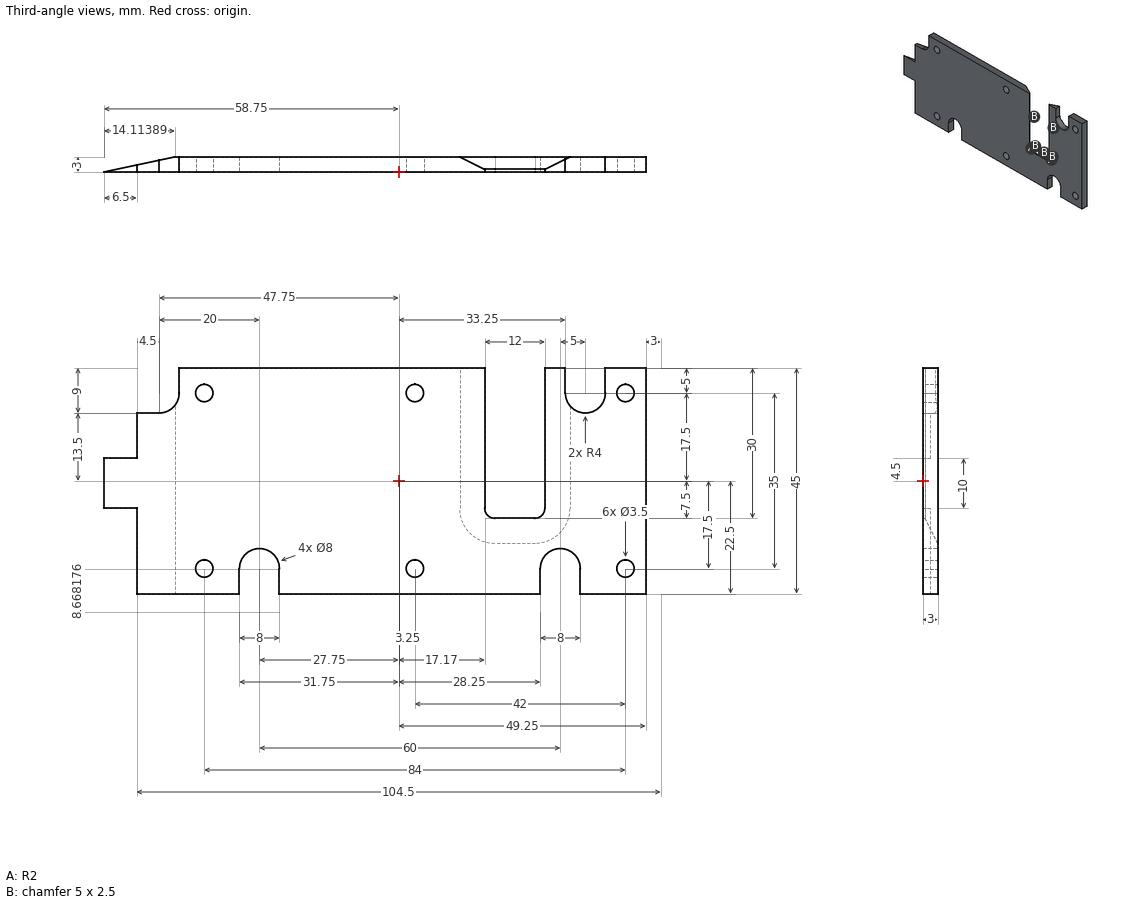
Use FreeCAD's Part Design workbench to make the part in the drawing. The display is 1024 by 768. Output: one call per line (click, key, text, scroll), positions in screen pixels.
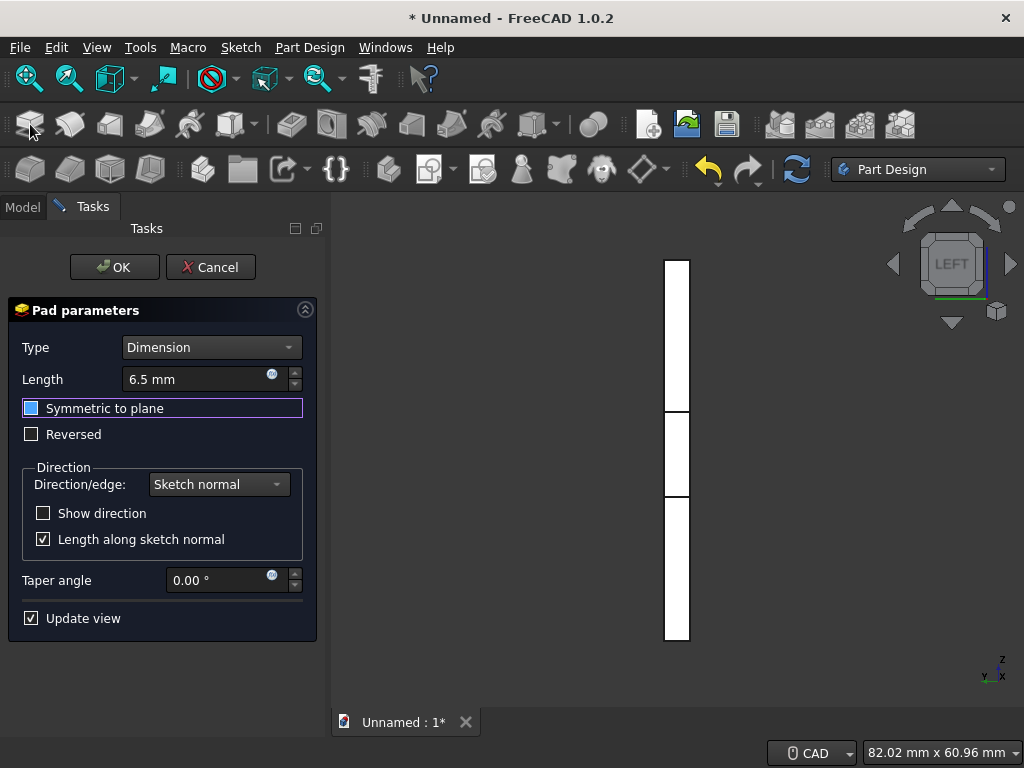
click(115, 267)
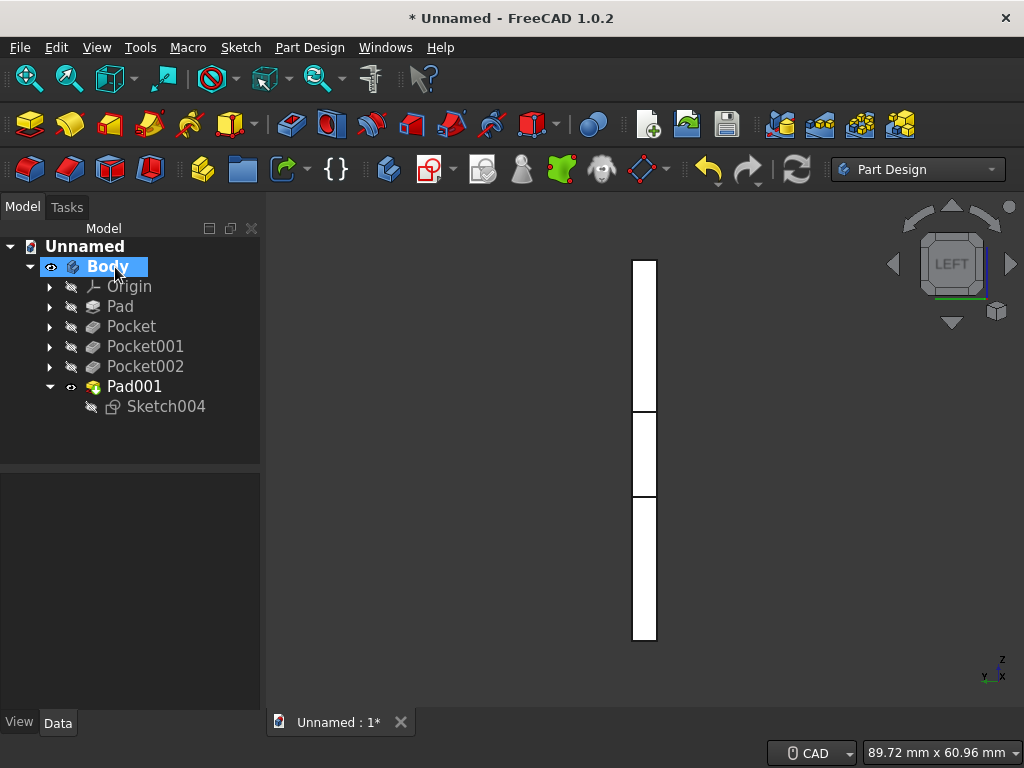
key(0)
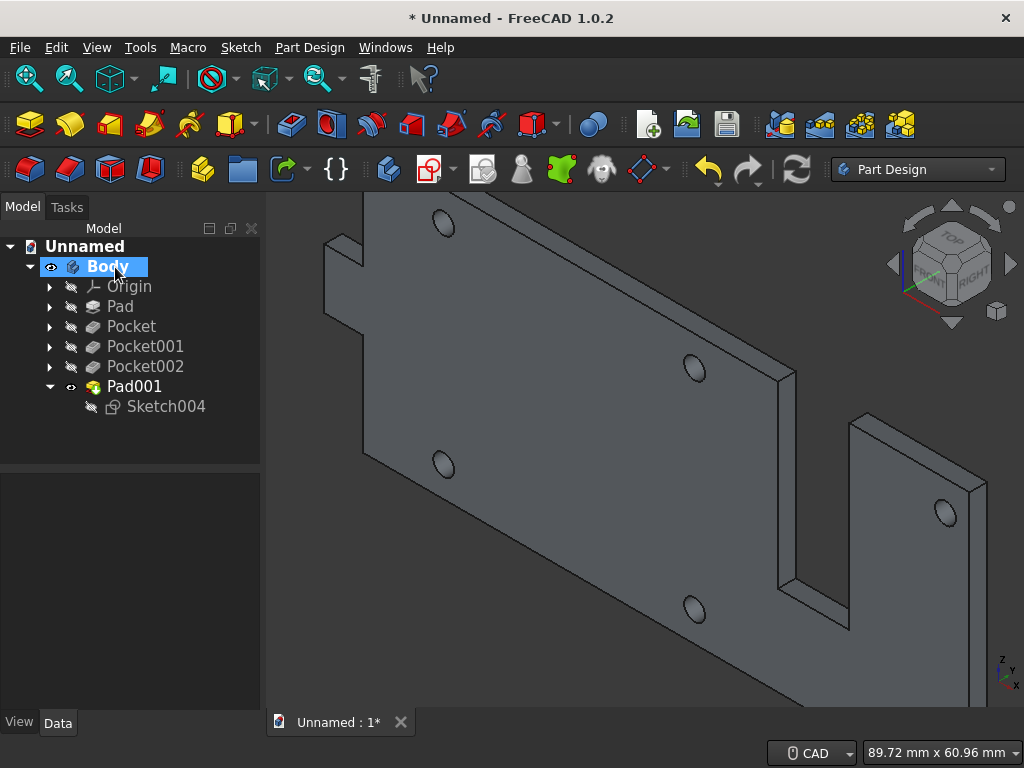
key(v)
key(f)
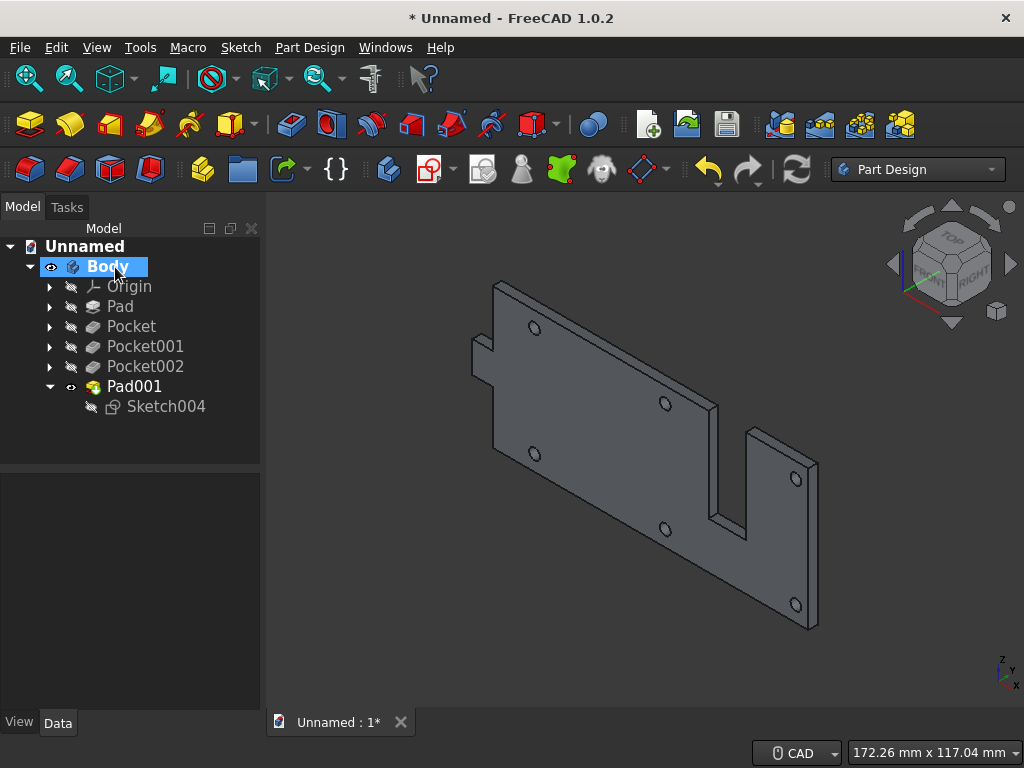
scroll(698, 398, up, 3)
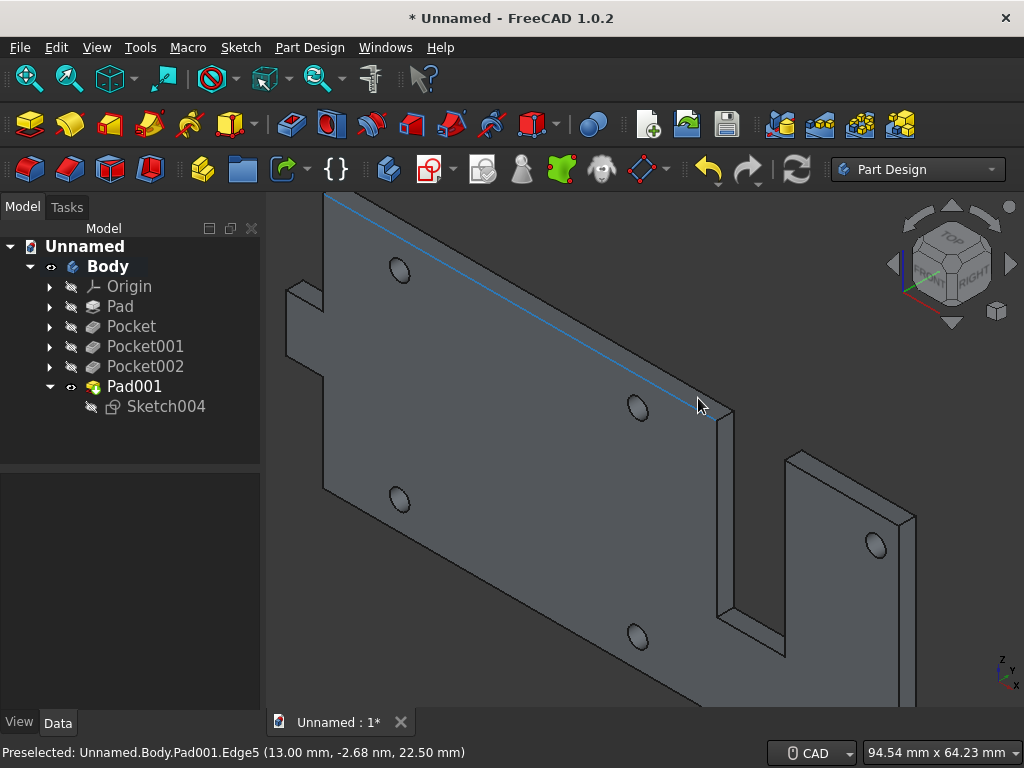
click(700, 397)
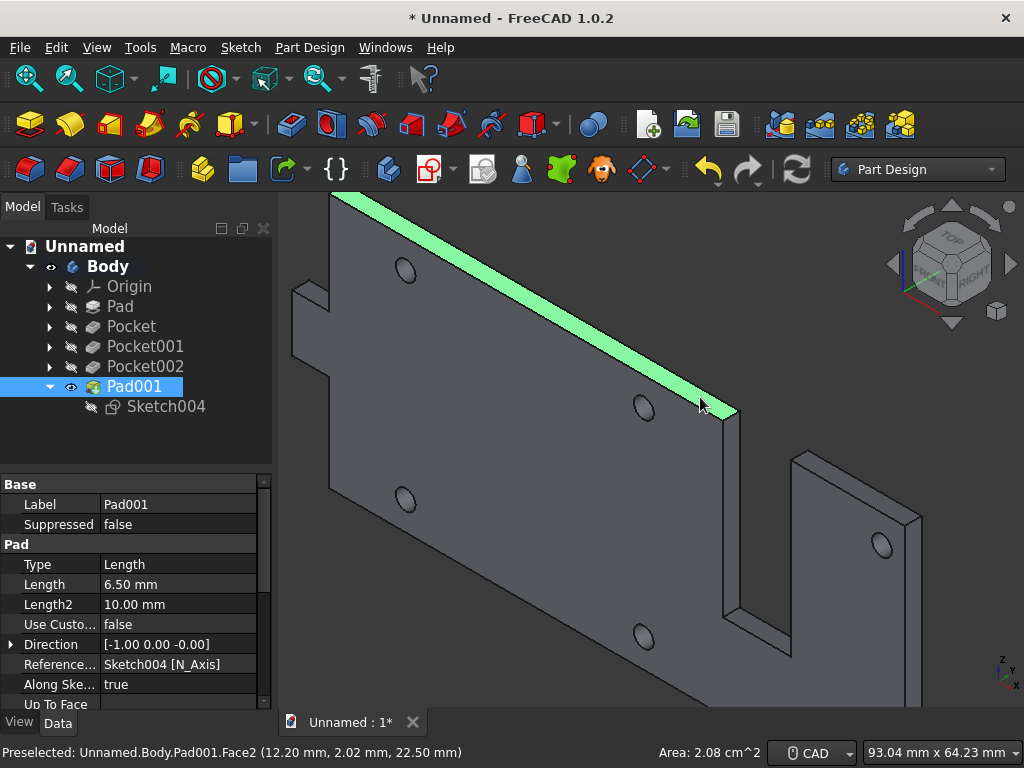
click(430, 170)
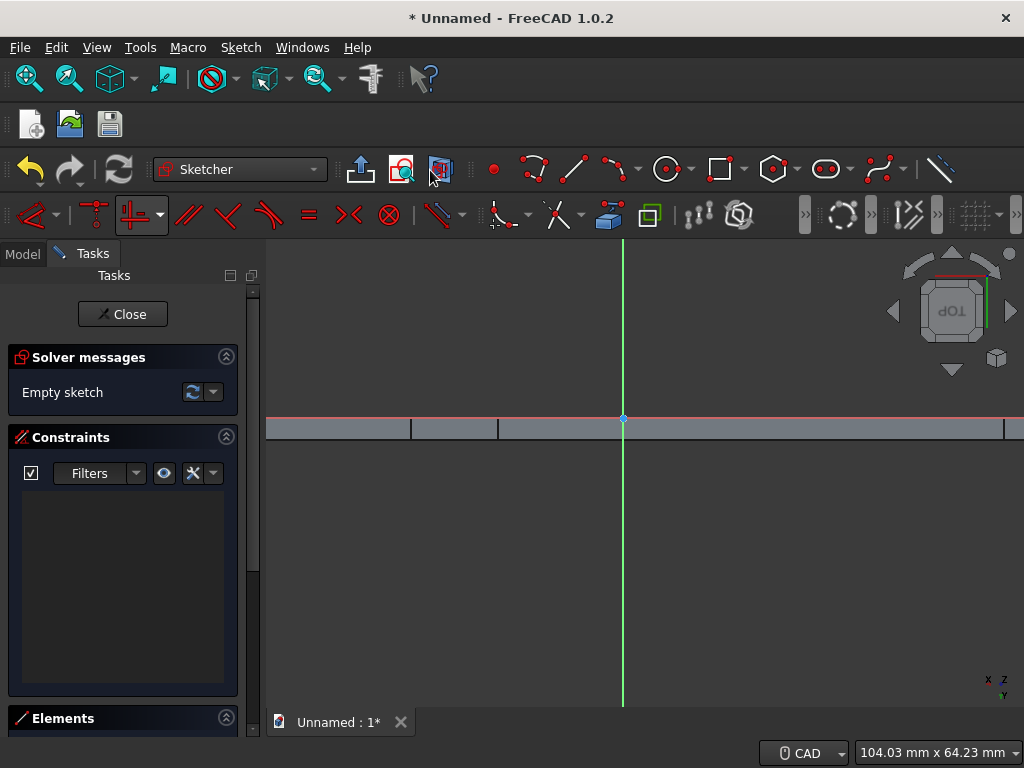
scroll(576, 473, down, 5)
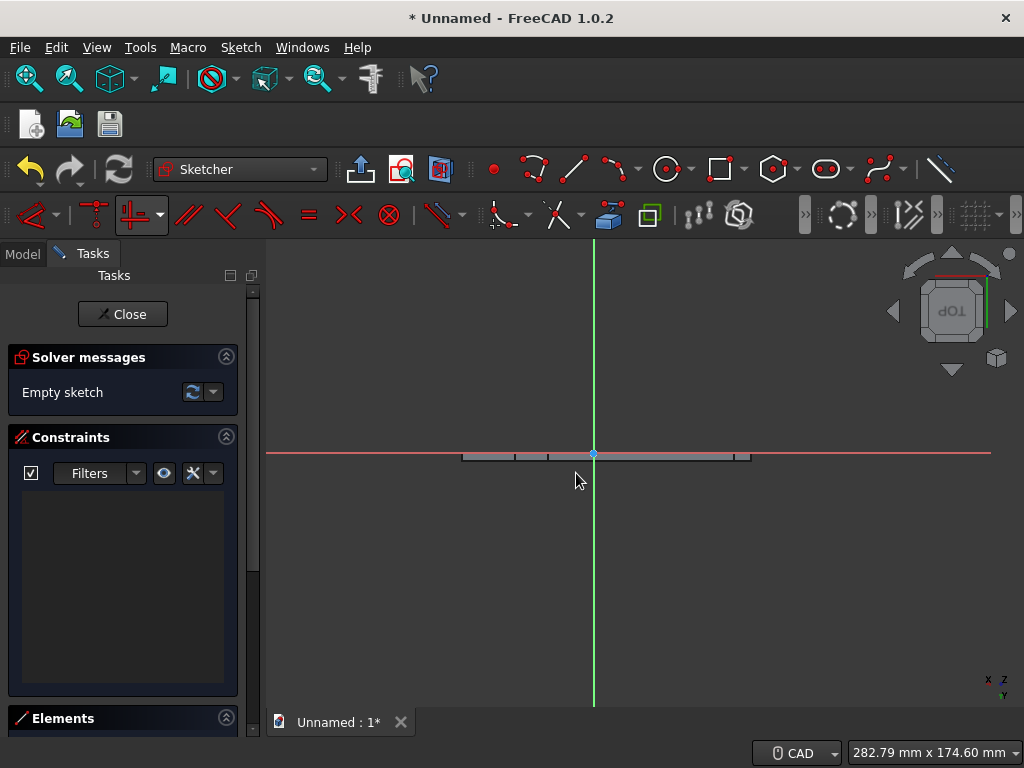
scroll(748, 456, up, 12)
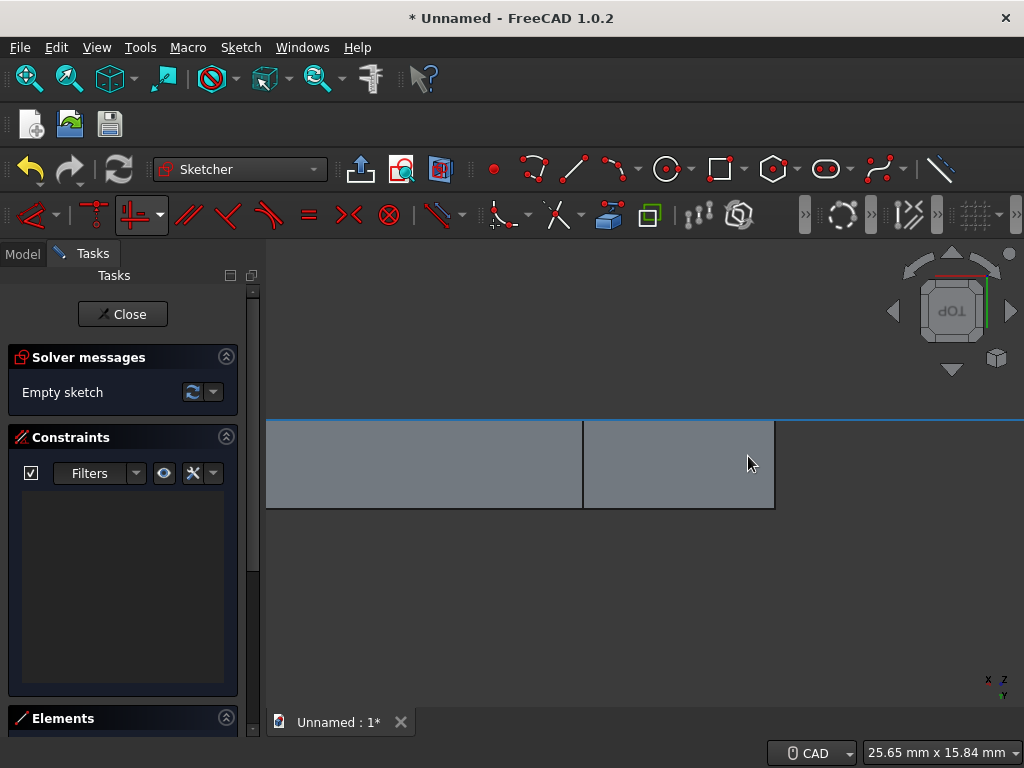
key(g)
key(m)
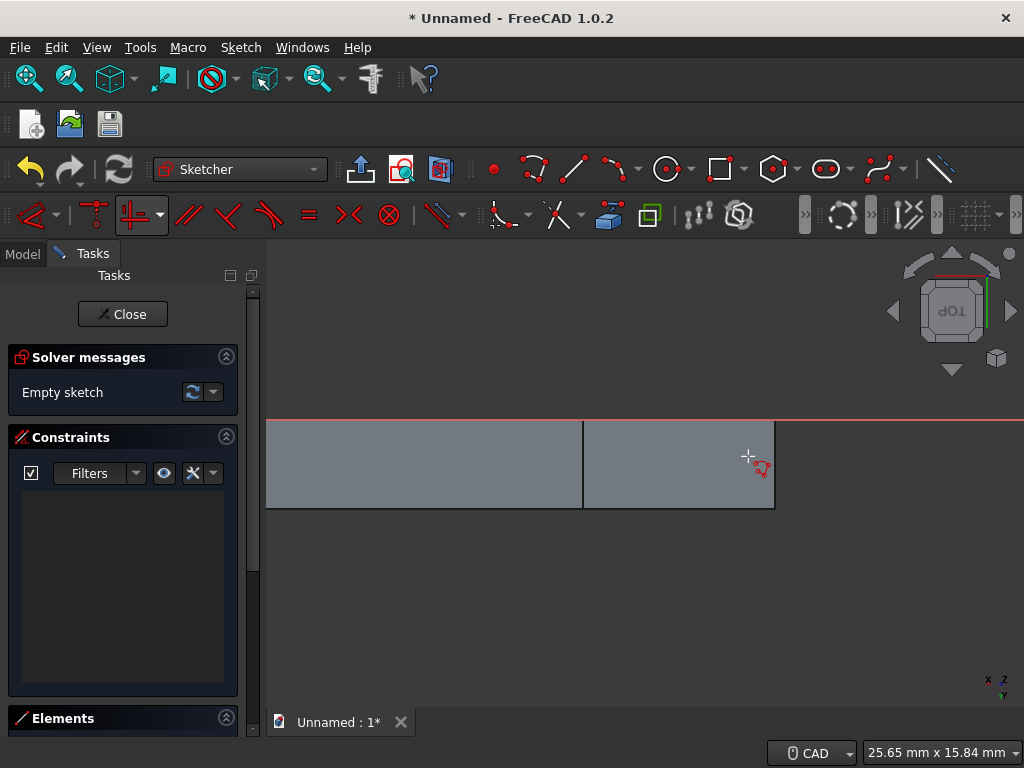
click(358, 509)
click(775, 509)
click(775, 420)
click(358, 510)
key(Escape)
key(Escape)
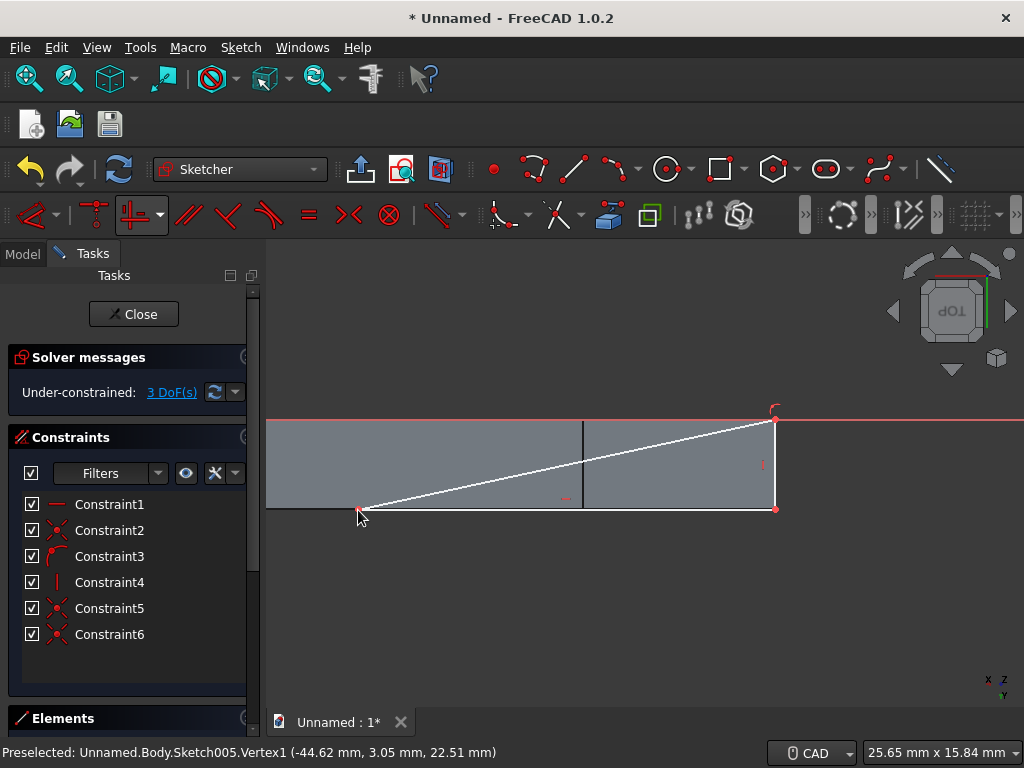
key(d)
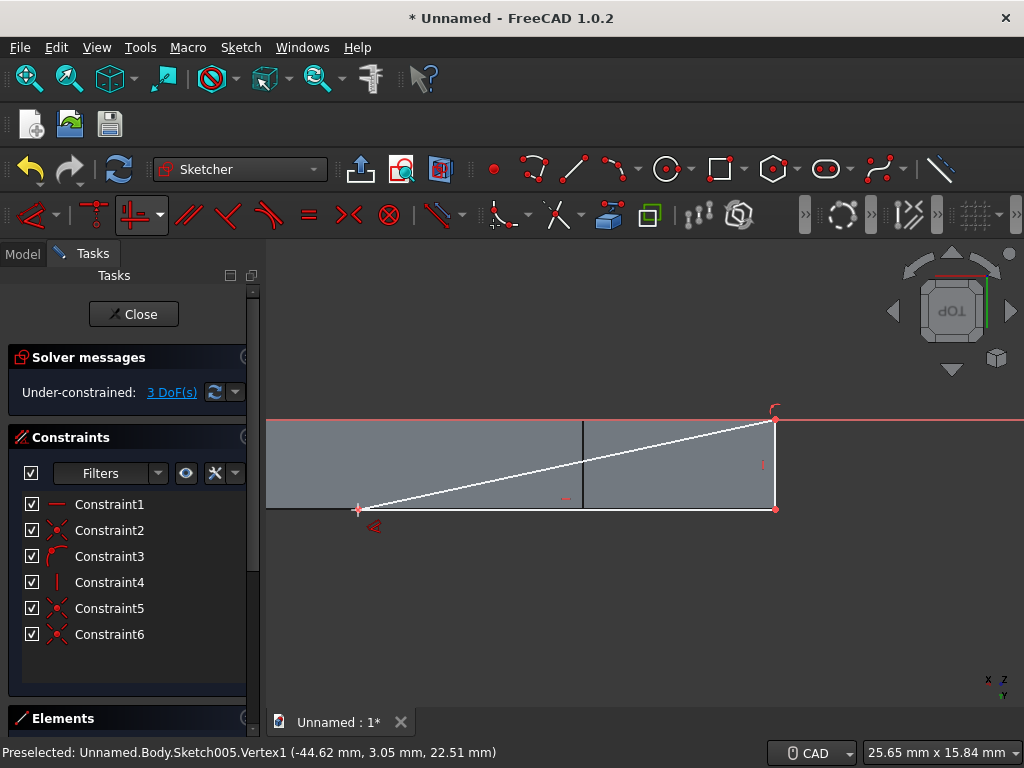
click(775, 483)
click(809, 465)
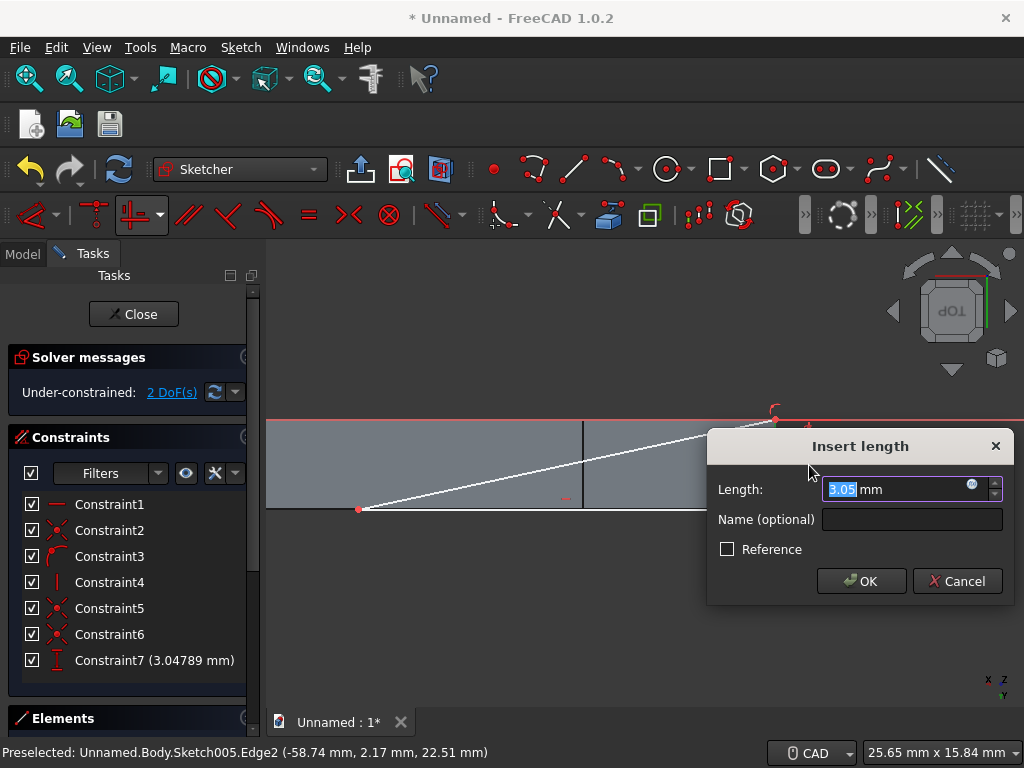
text(3)
key(Return)